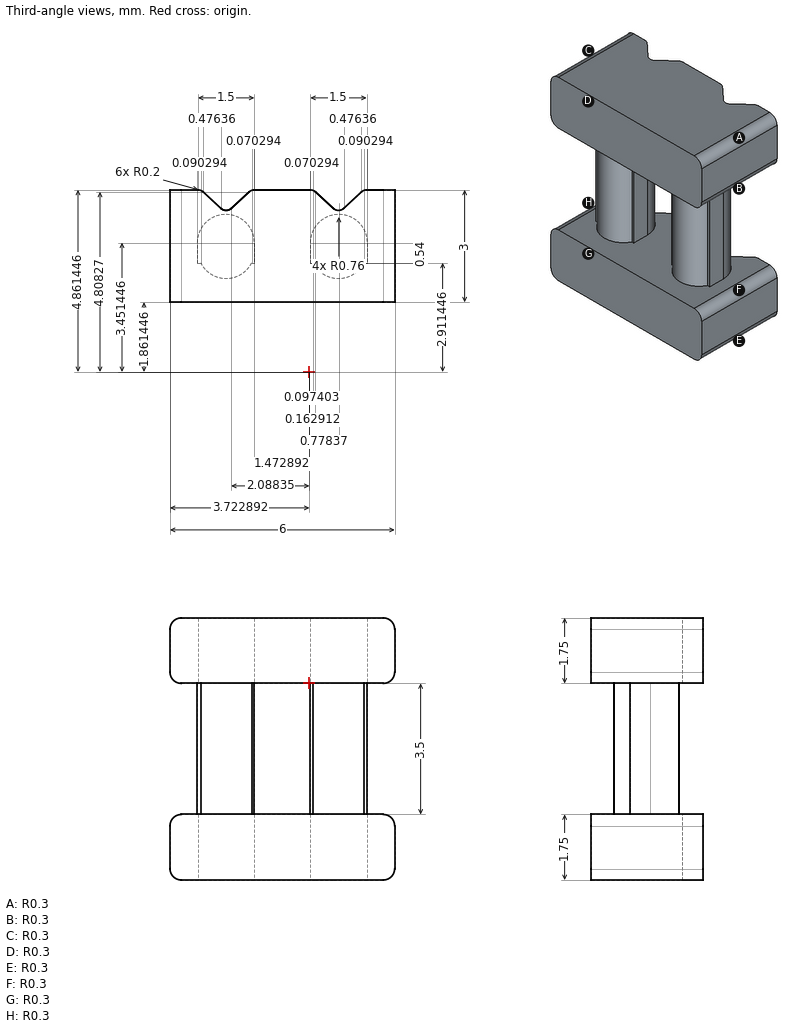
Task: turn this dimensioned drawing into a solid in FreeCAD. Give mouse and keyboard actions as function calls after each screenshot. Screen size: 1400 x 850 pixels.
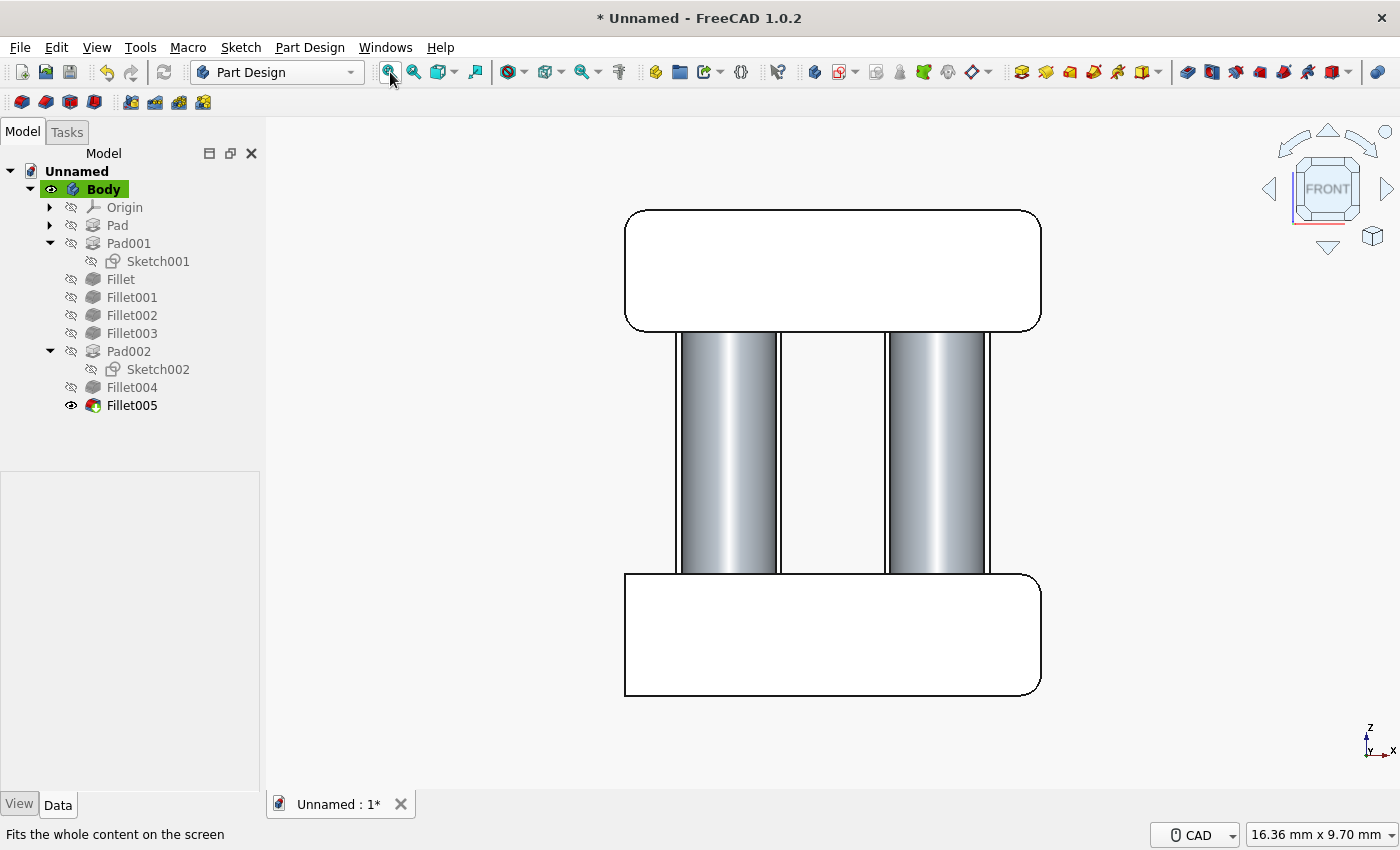
key(3)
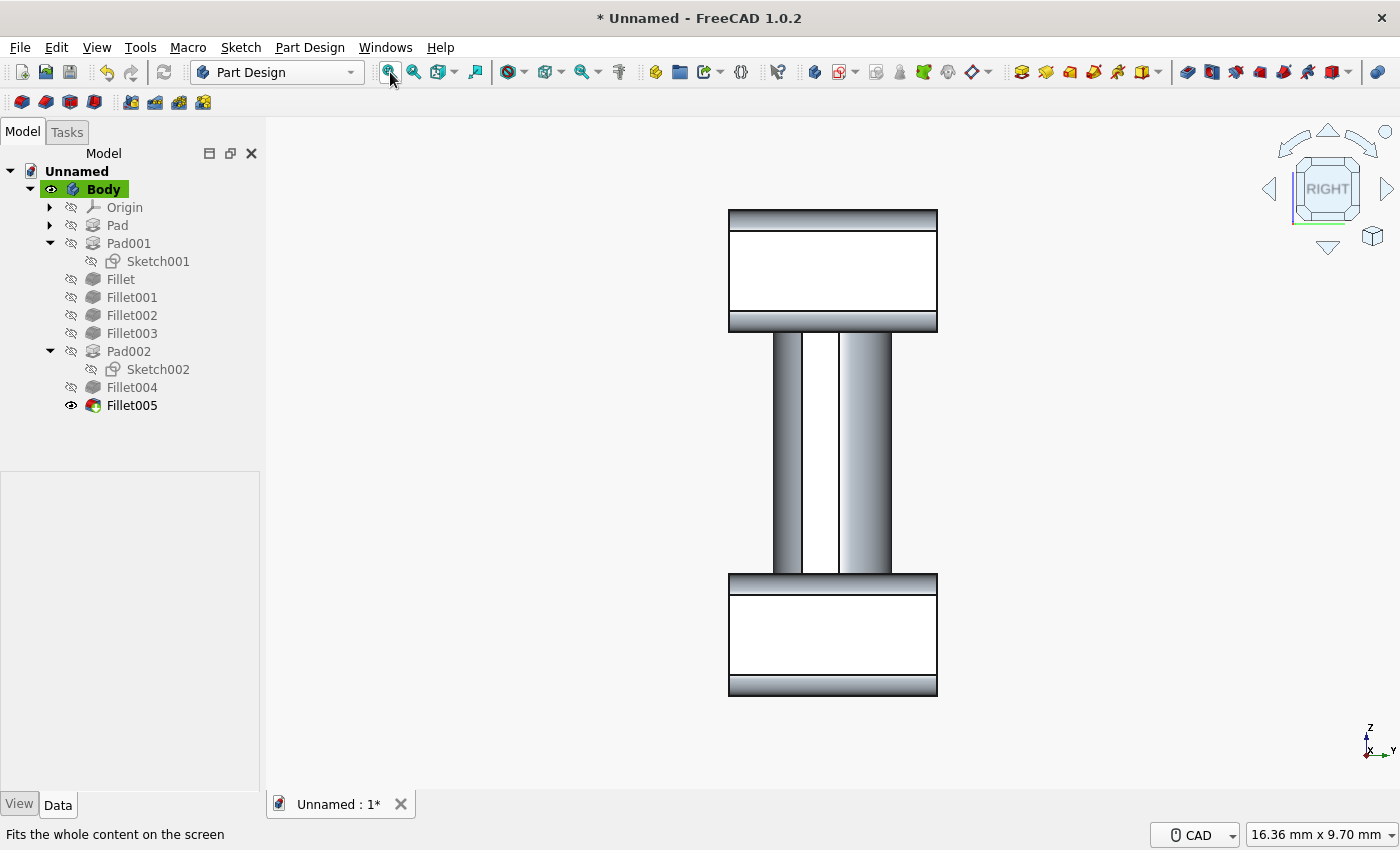
key(5)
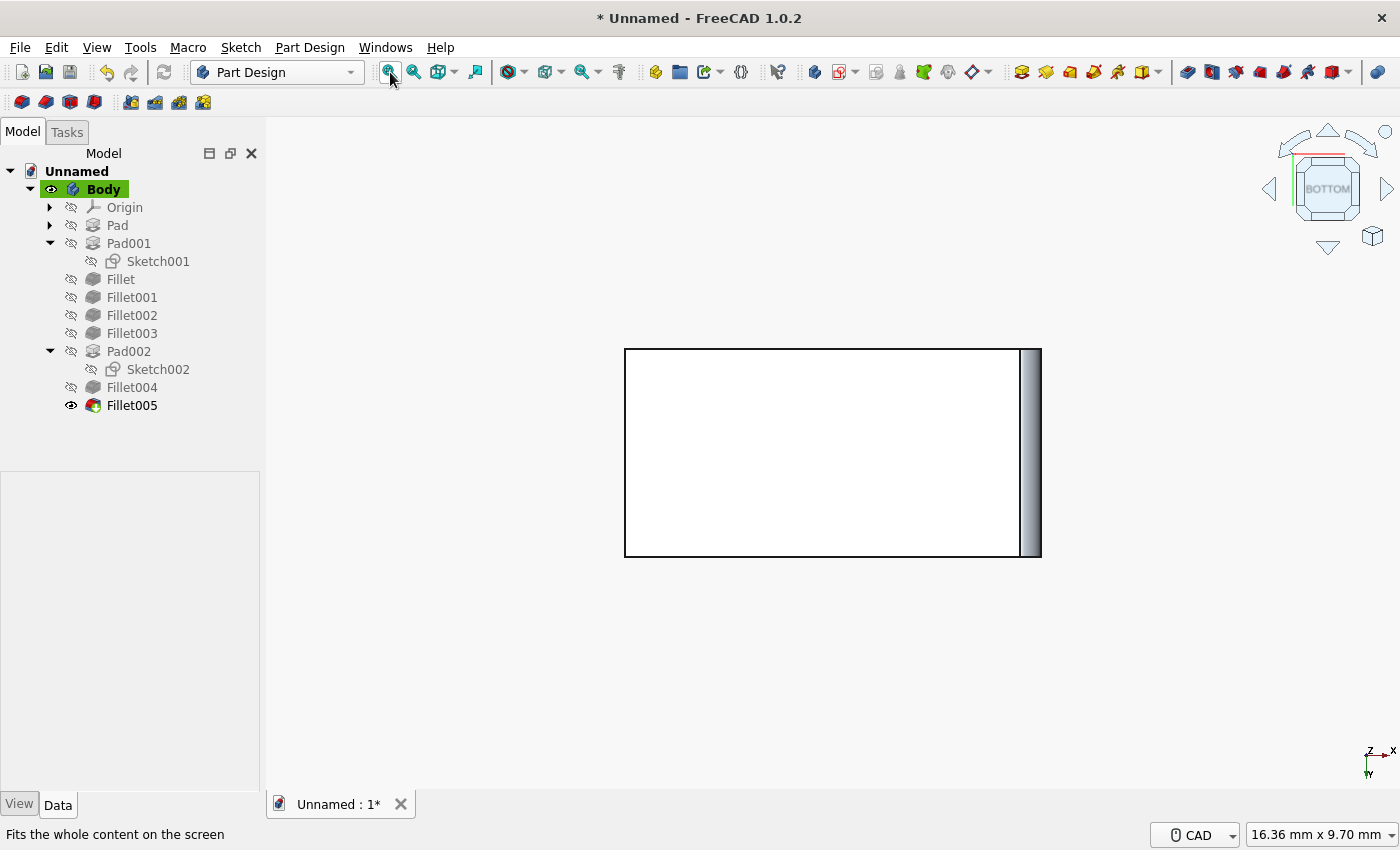
click(390, 72)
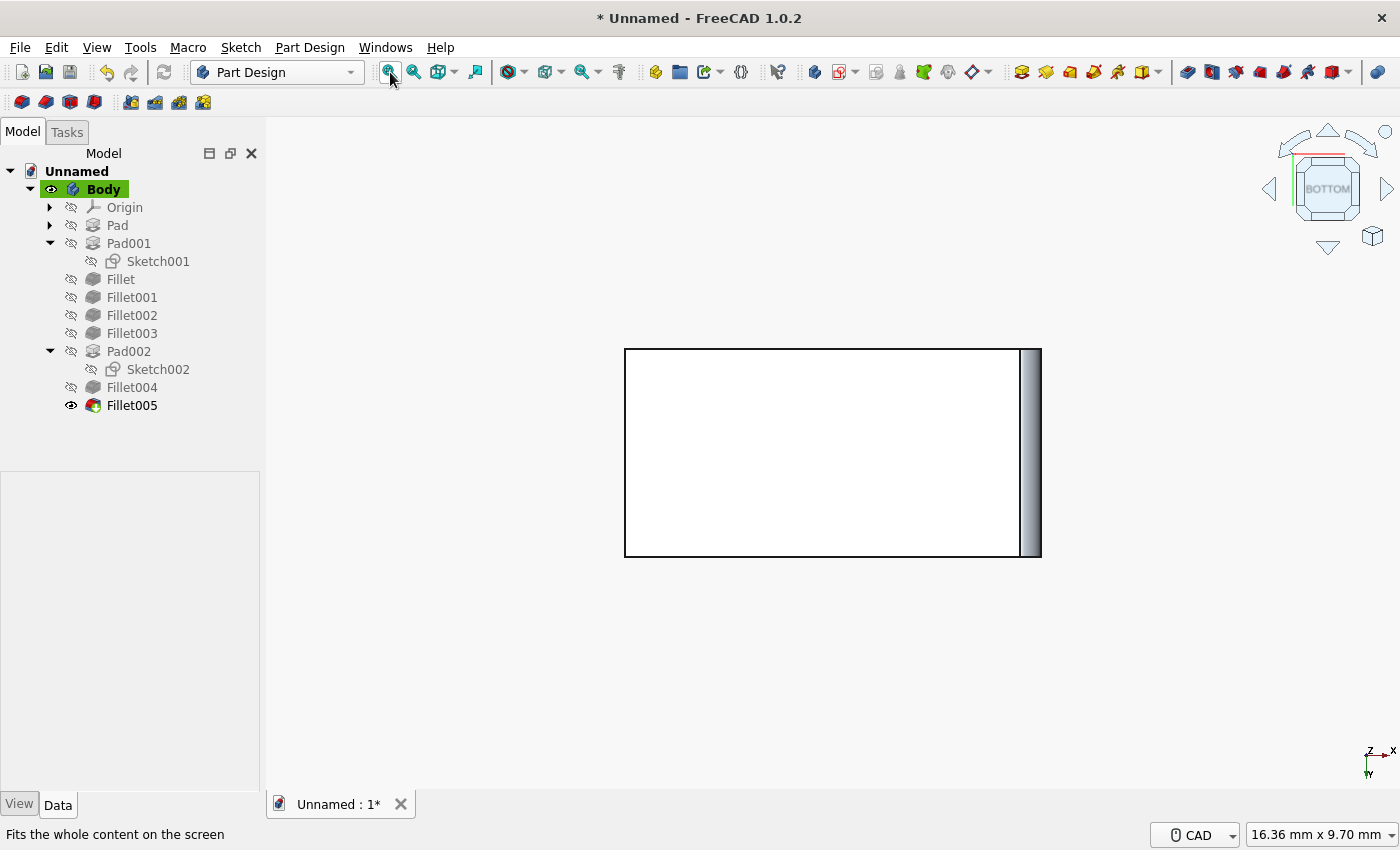
click(625, 452)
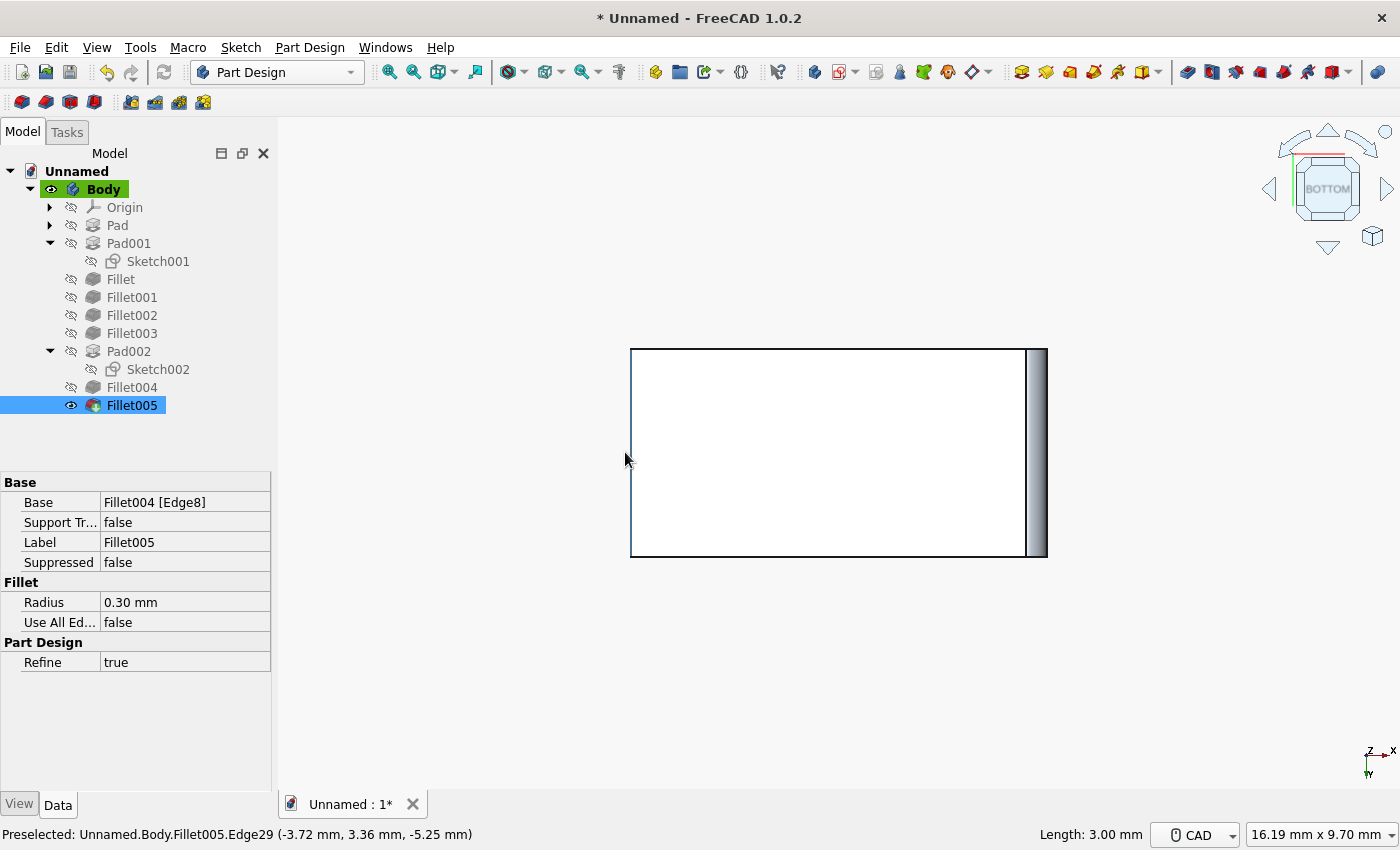
click(22, 102)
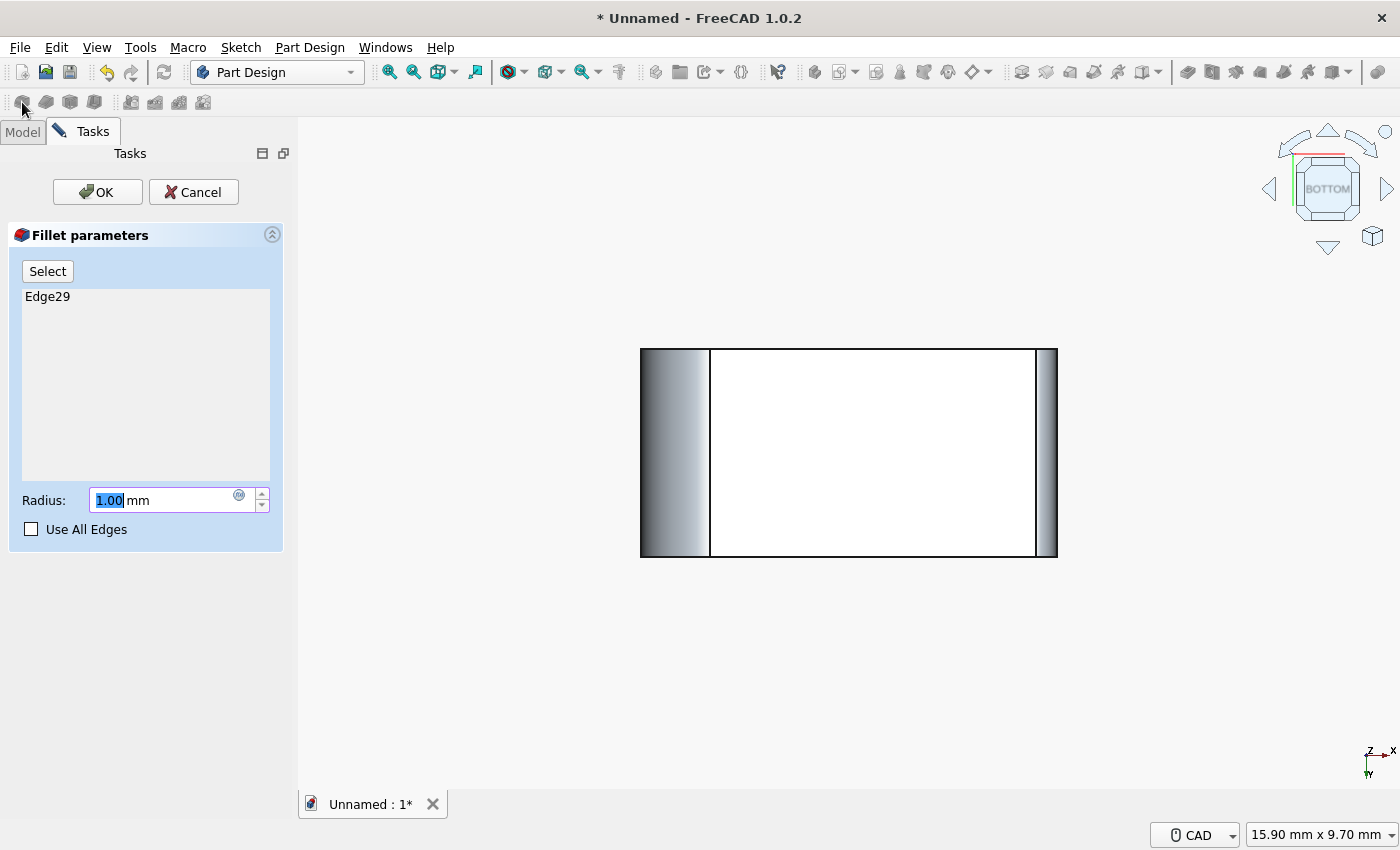
text(0.3)
key(Tab)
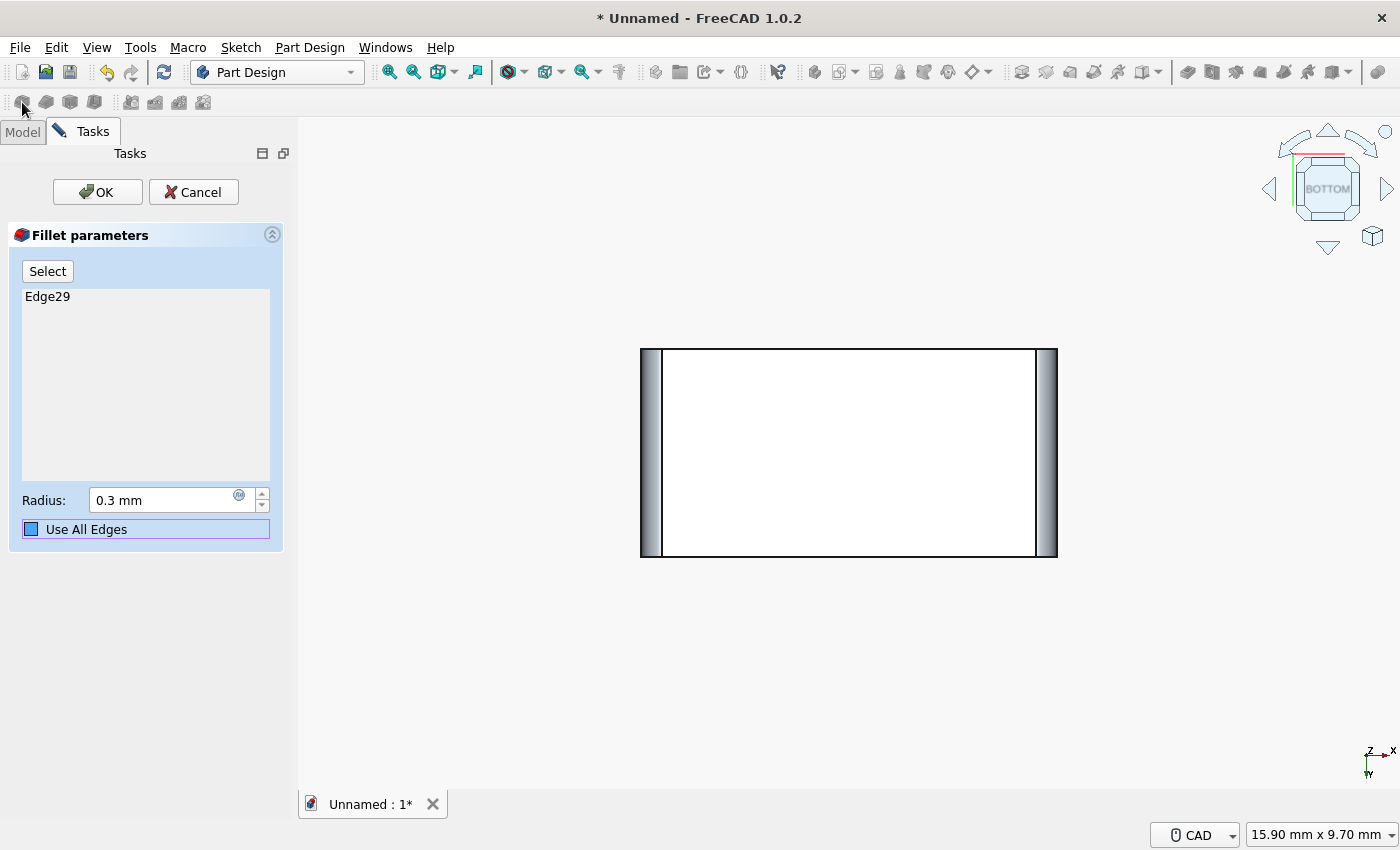
click(98, 192)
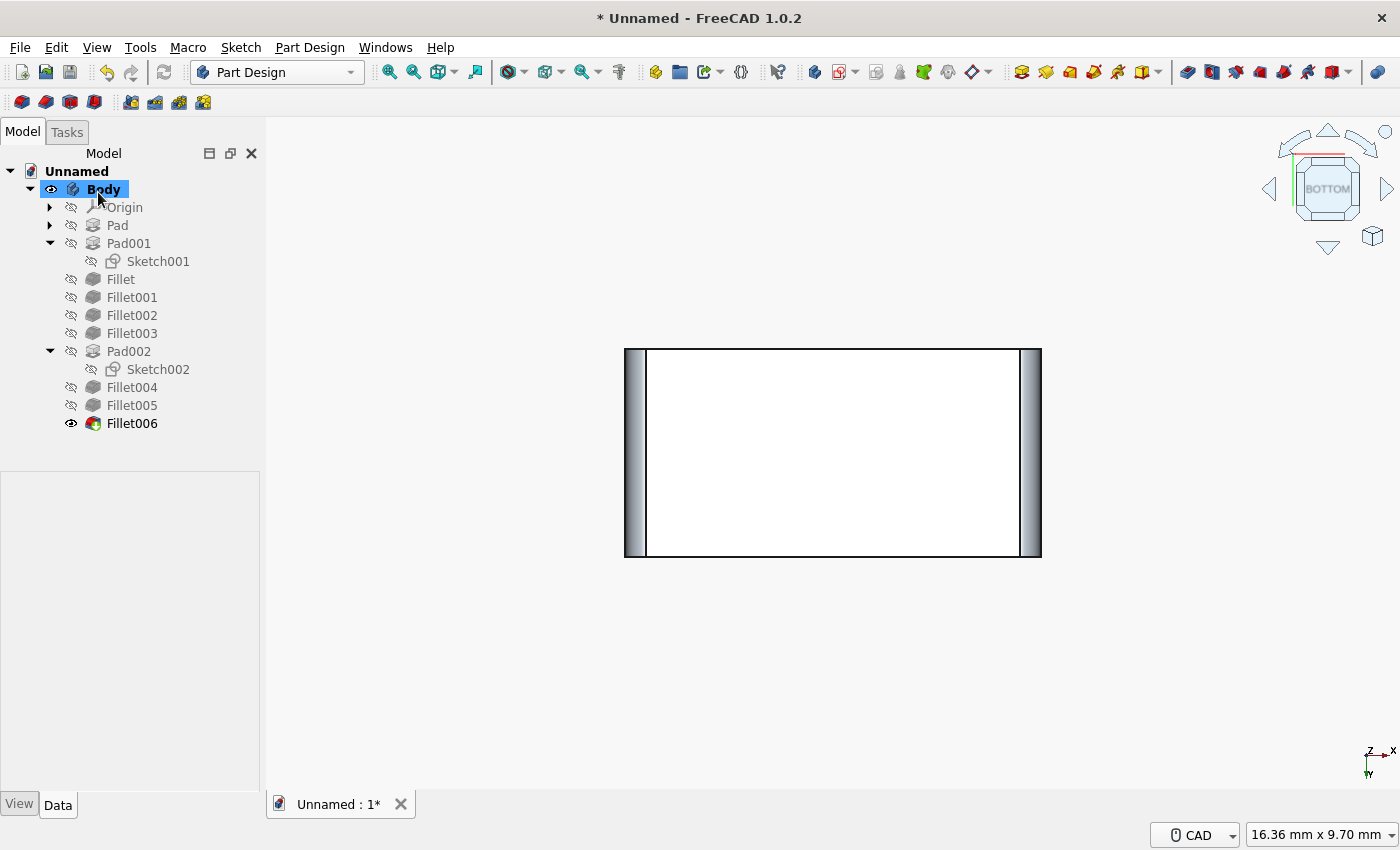
click(390, 72)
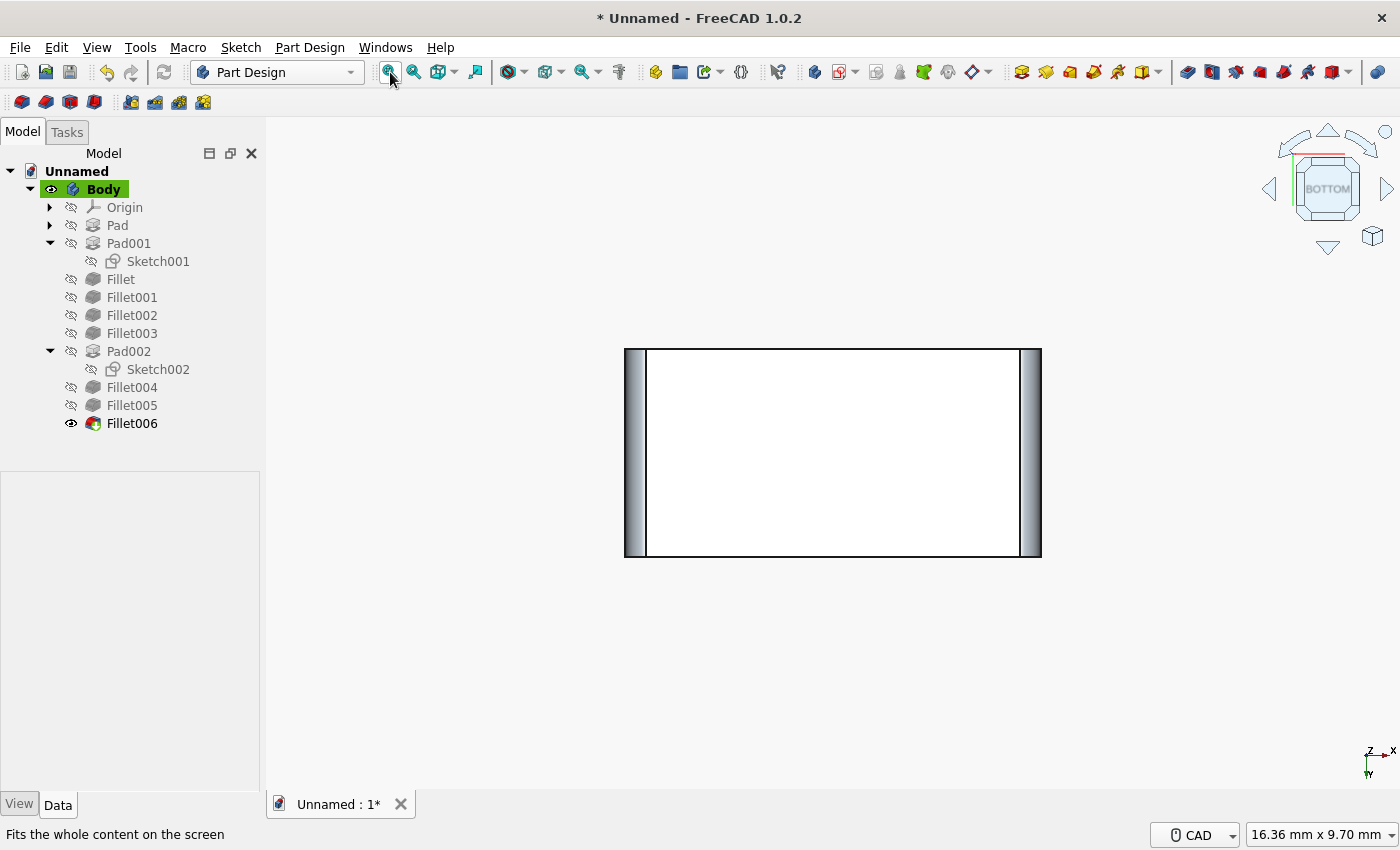
key(0)